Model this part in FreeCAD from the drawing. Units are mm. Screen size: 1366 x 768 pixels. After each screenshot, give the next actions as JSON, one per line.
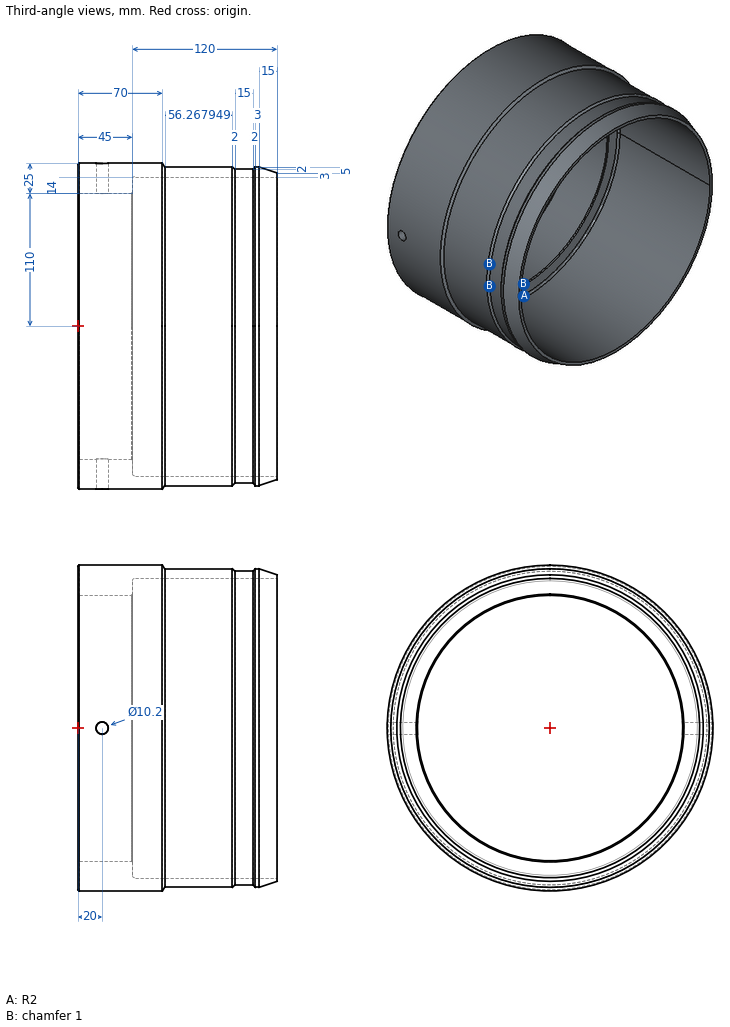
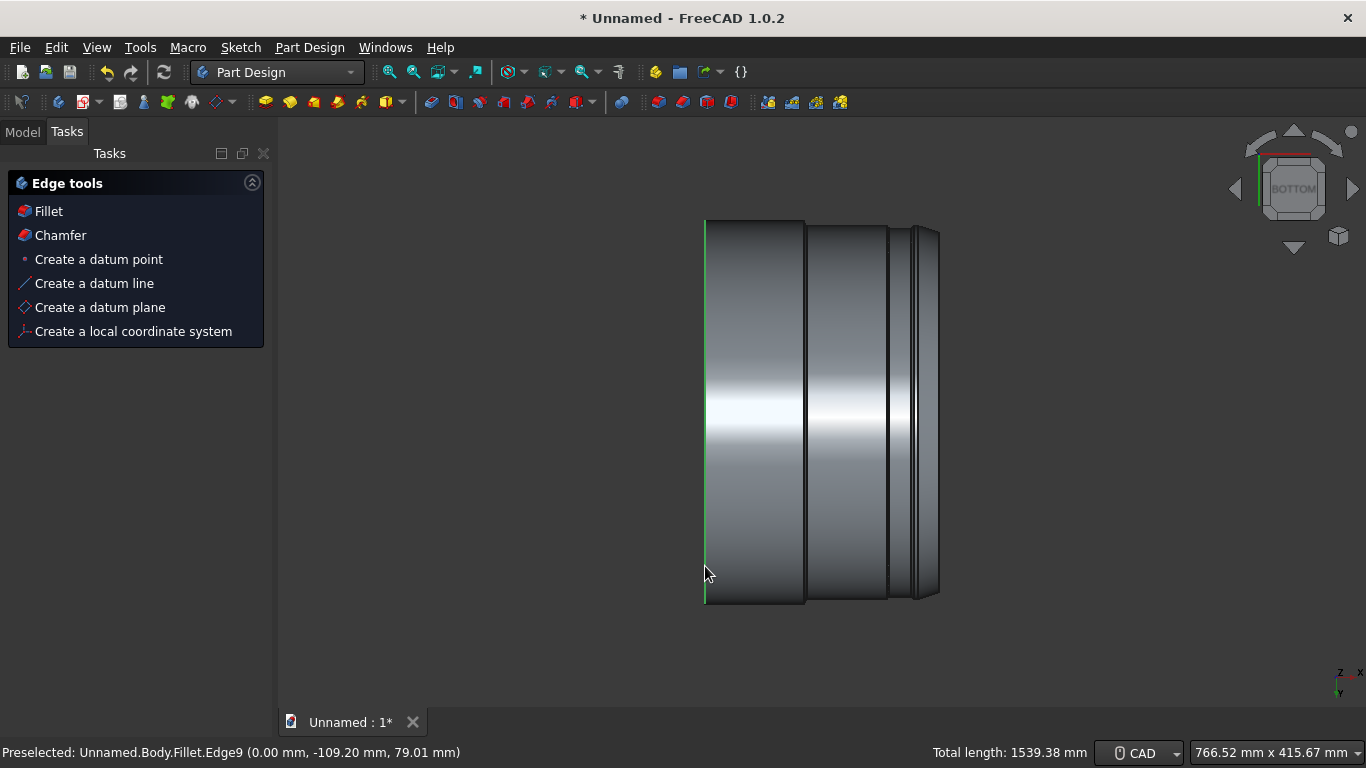
{"action": "key", "text": "4"}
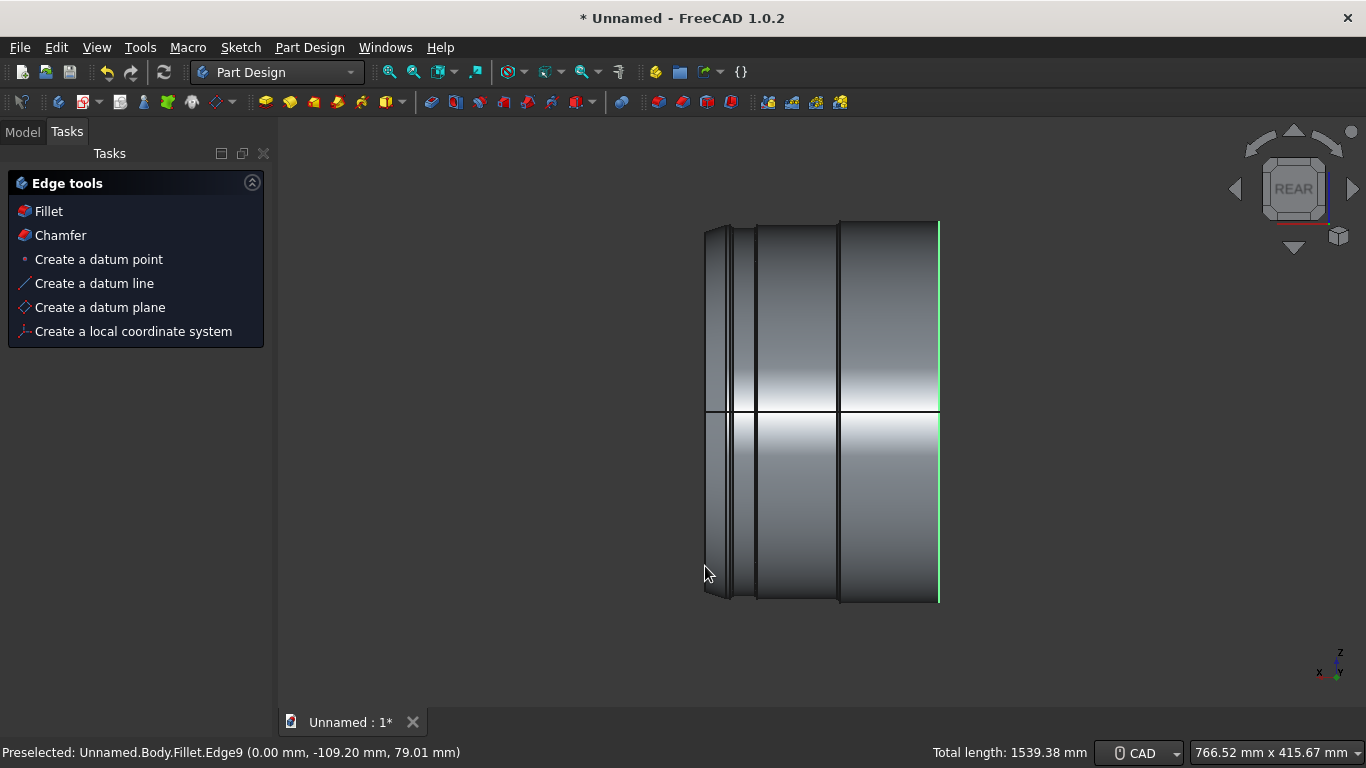
{"action": "key", "text": "6"}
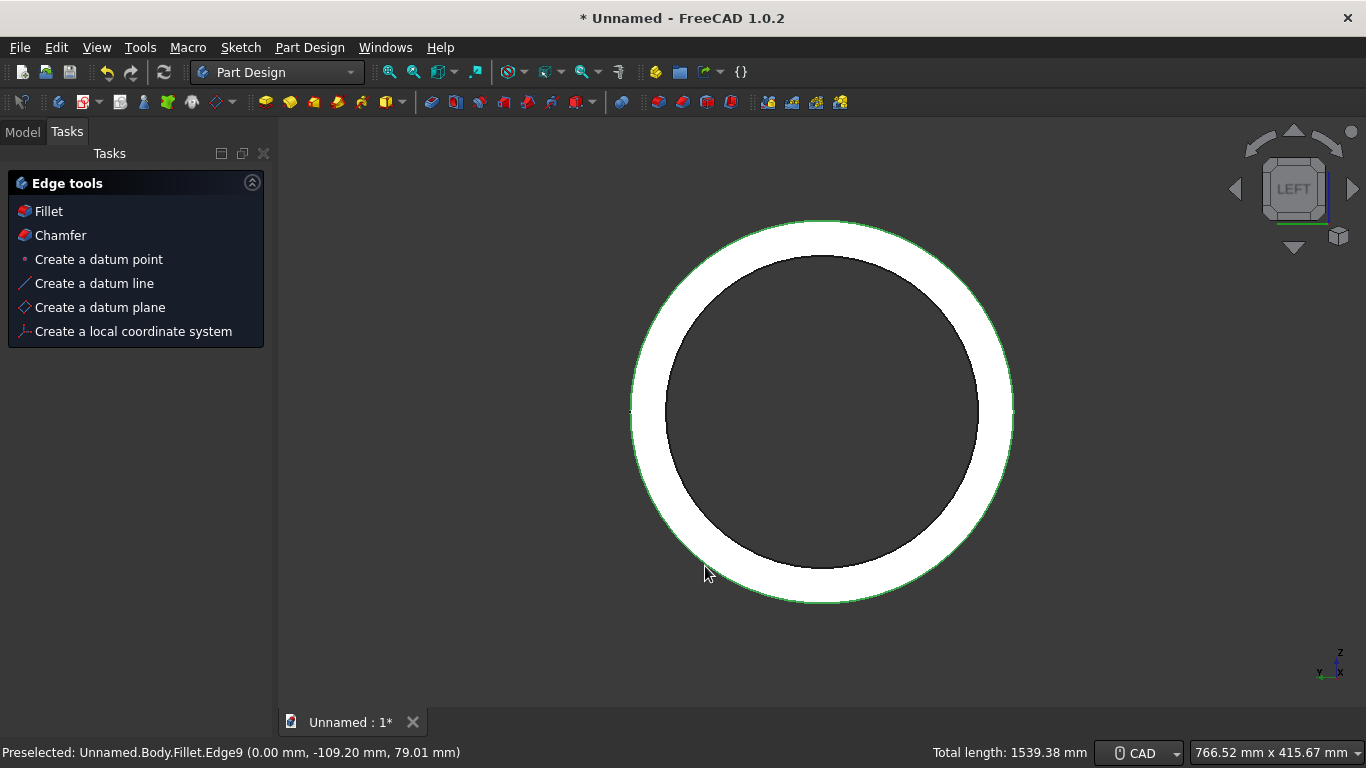
{"action": "left_click", "coordinate": [978, 411], "text": "ctrl"}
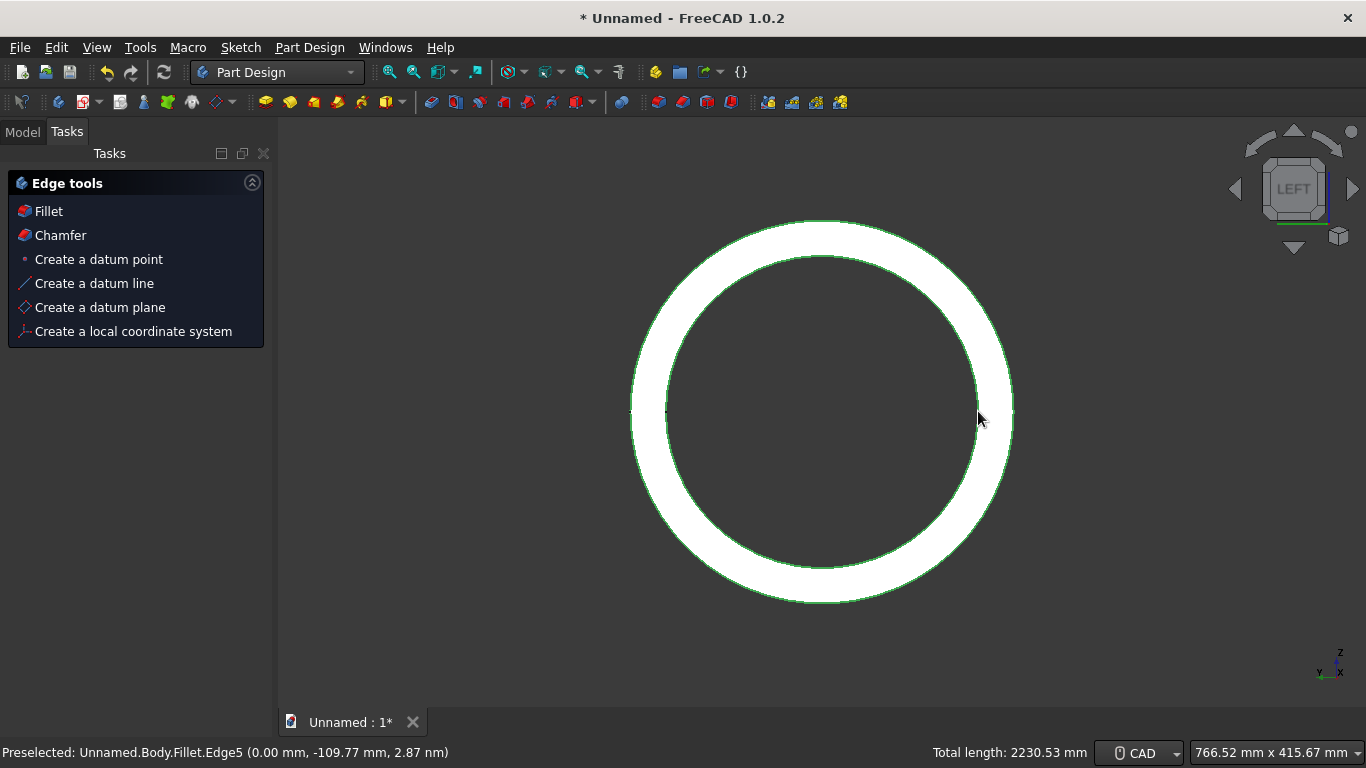
{"action": "left_click", "coordinate": [684, 102]}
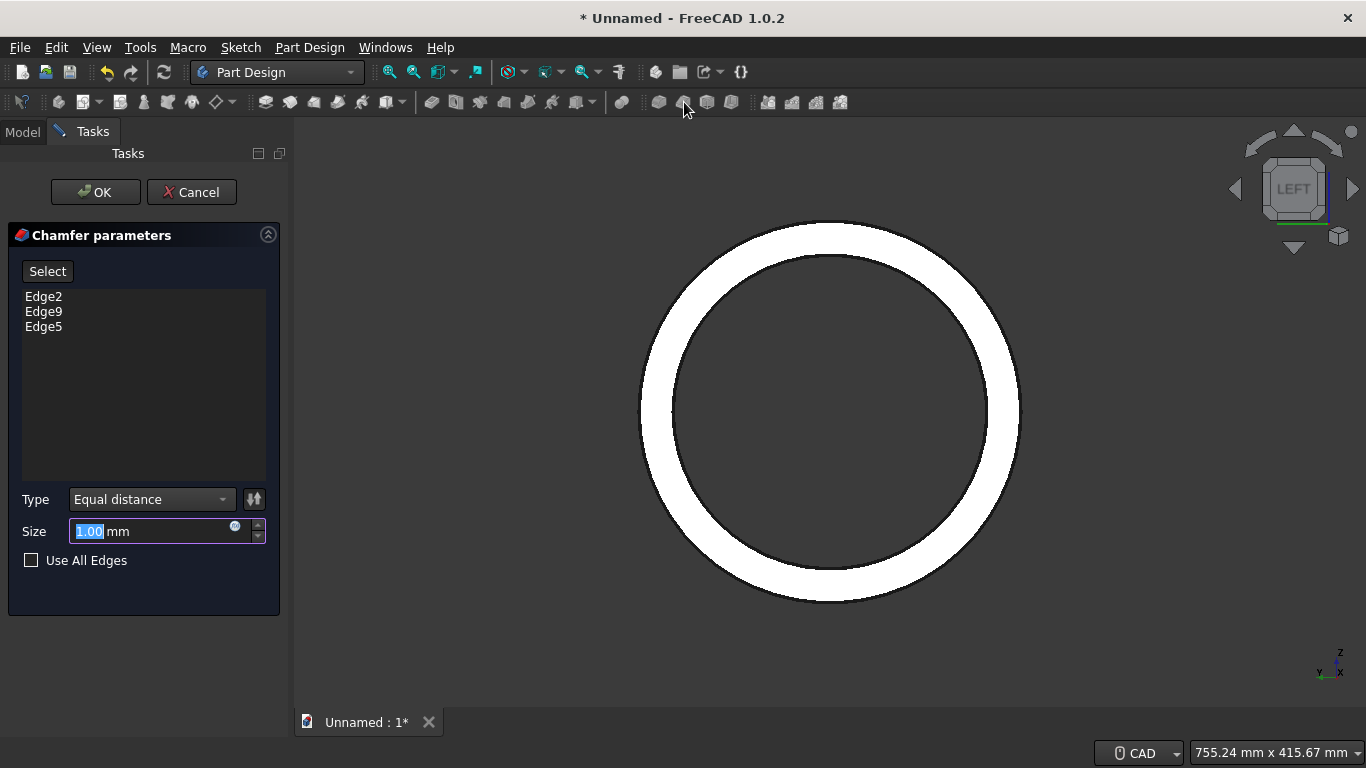
{"action": "type", "text": "1"}
{"action": "key", "text": "Tab"}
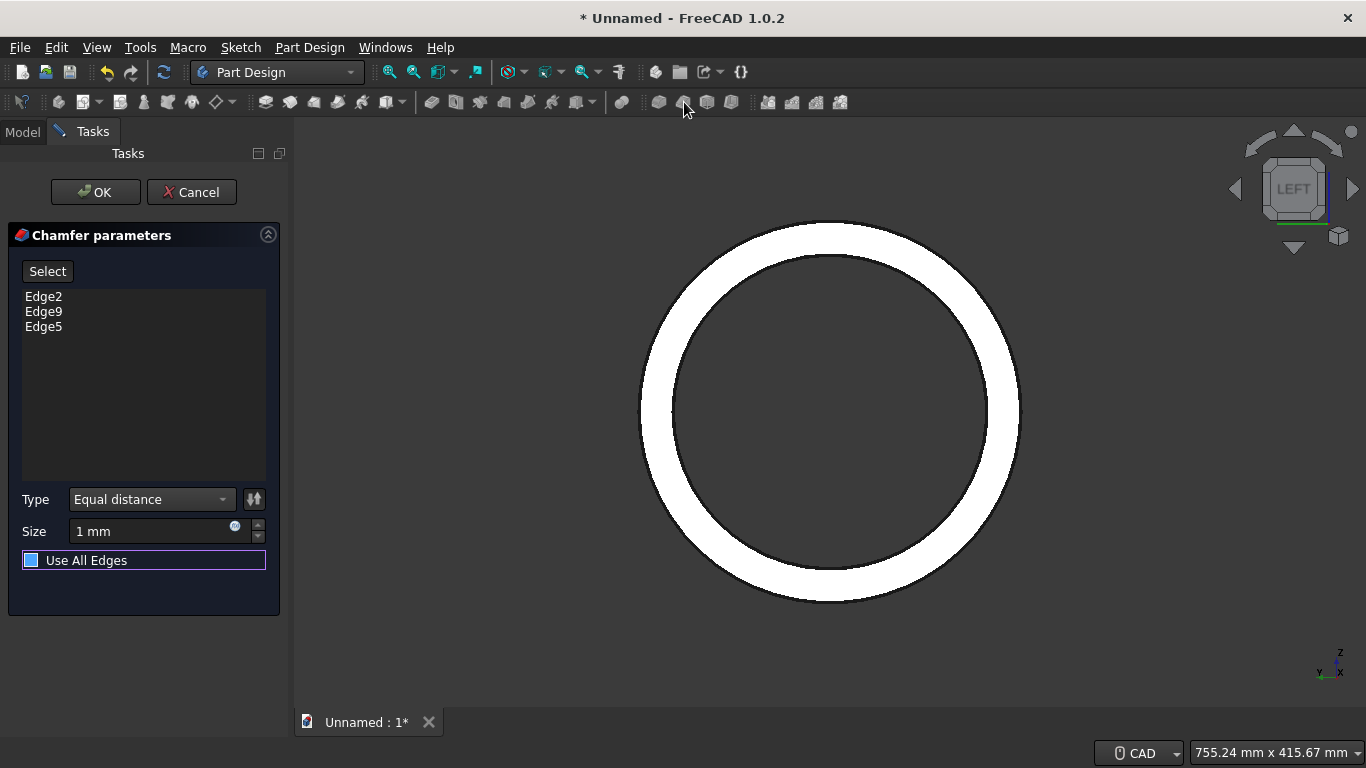
{"action": "left_click", "coordinate": [96, 192]}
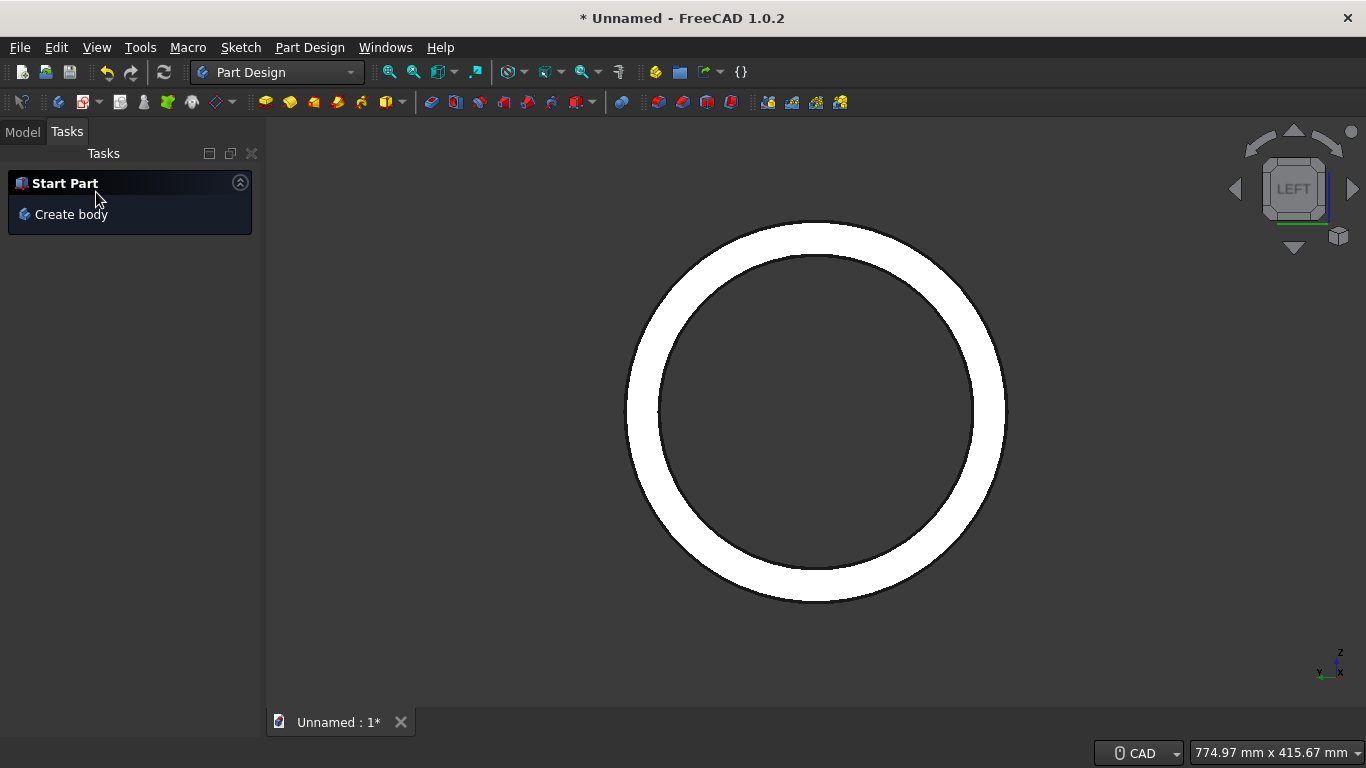
{"action": "left_click", "coordinate": [23, 131]}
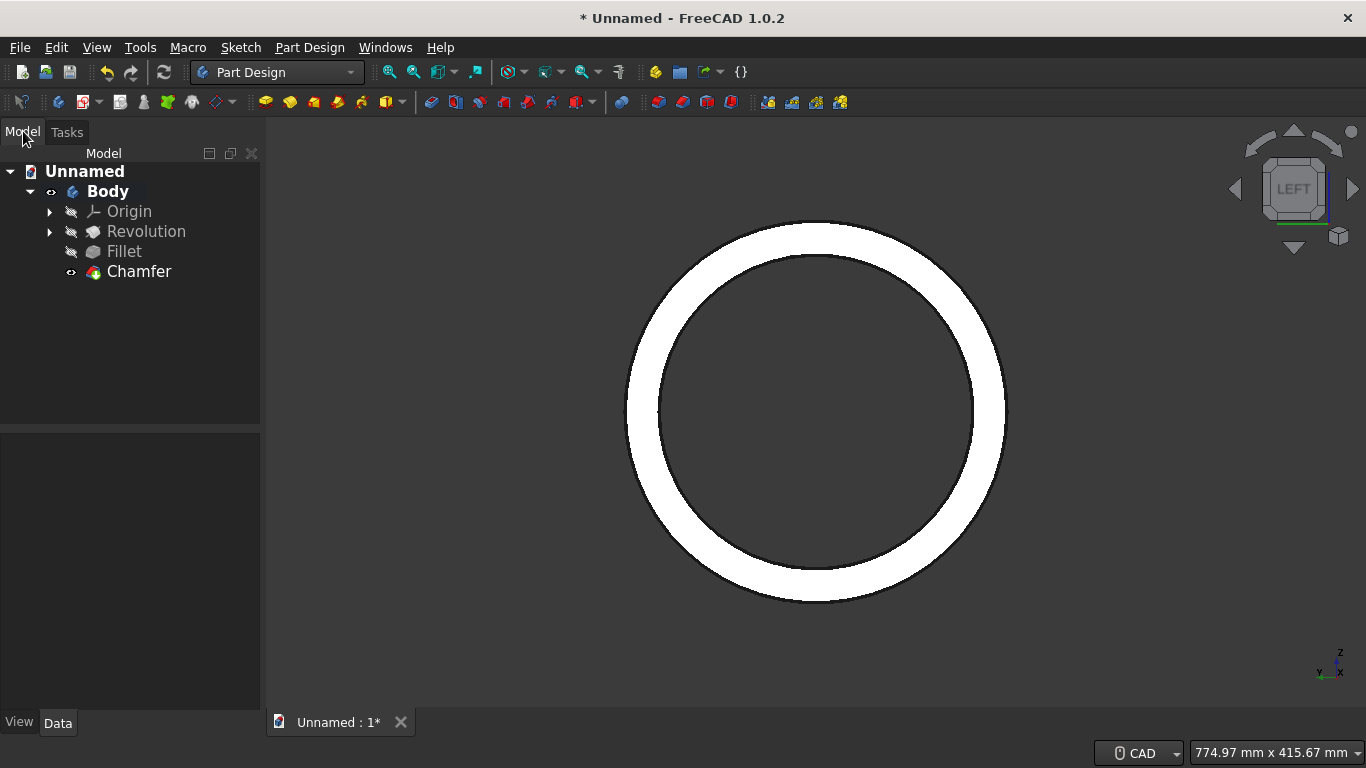
{"action": "left_click", "coordinate": [50, 212]}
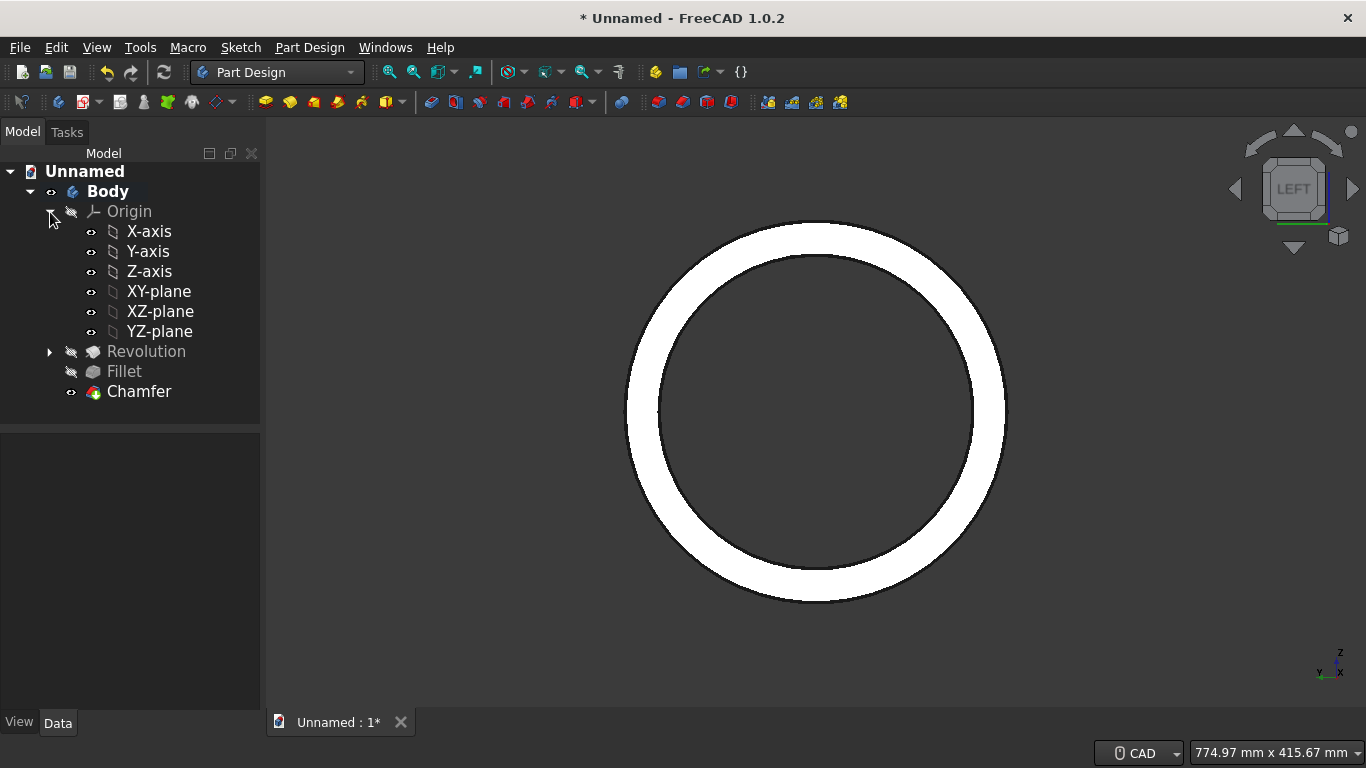
{"action": "left_click", "coordinate": [136, 312]}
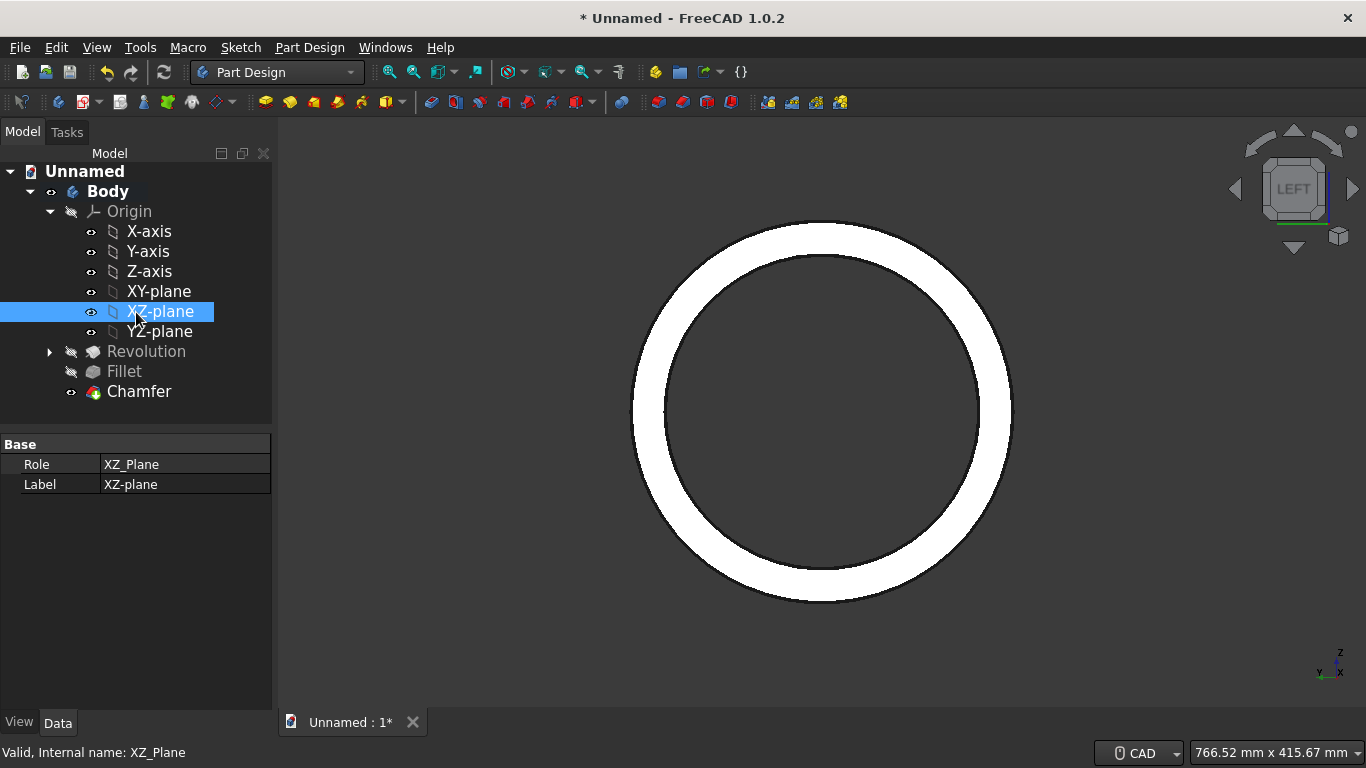
{"action": "left_click", "coordinate": [216, 102]}